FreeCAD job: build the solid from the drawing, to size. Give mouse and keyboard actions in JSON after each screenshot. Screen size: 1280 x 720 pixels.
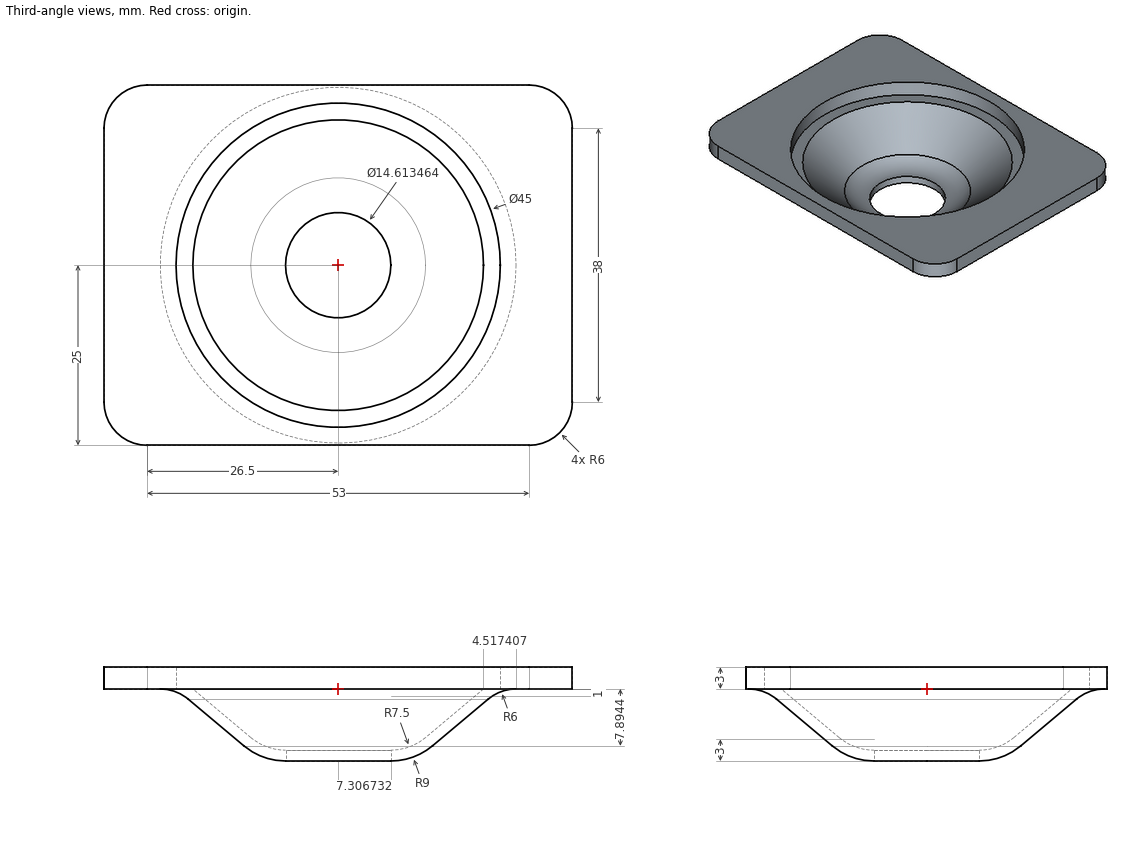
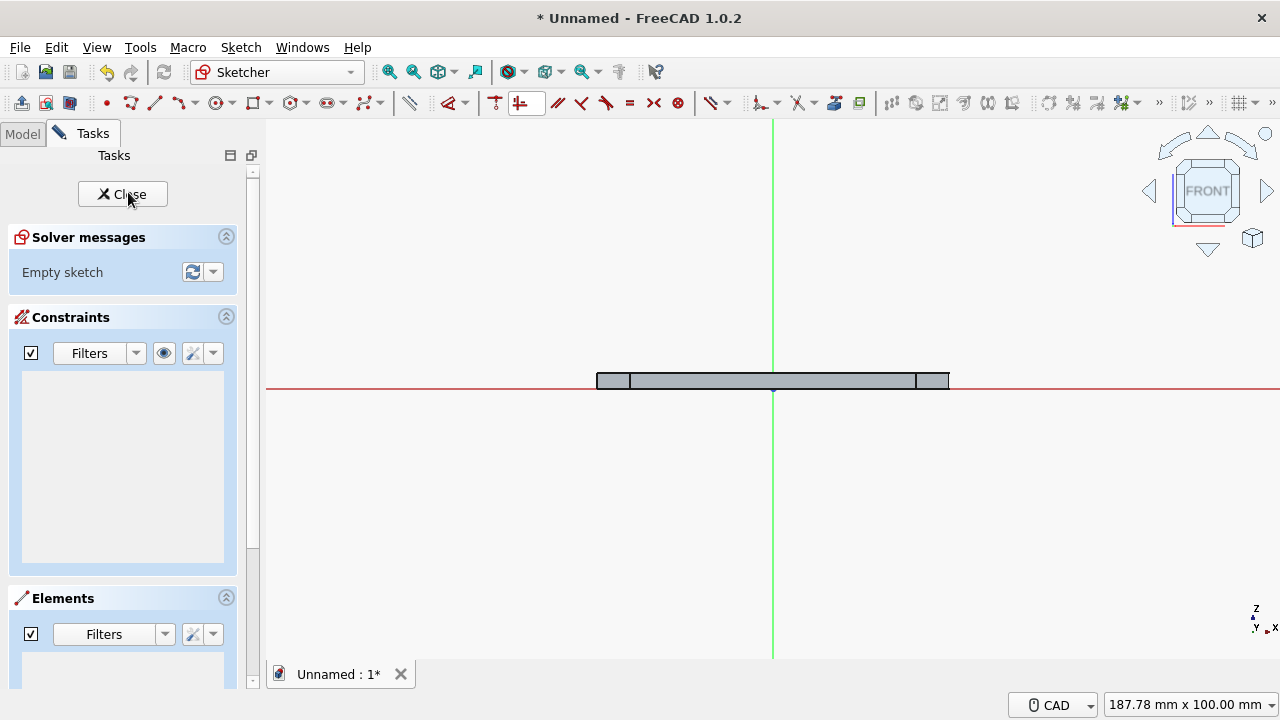
{"action": "left_click", "coordinate": [70, 104]}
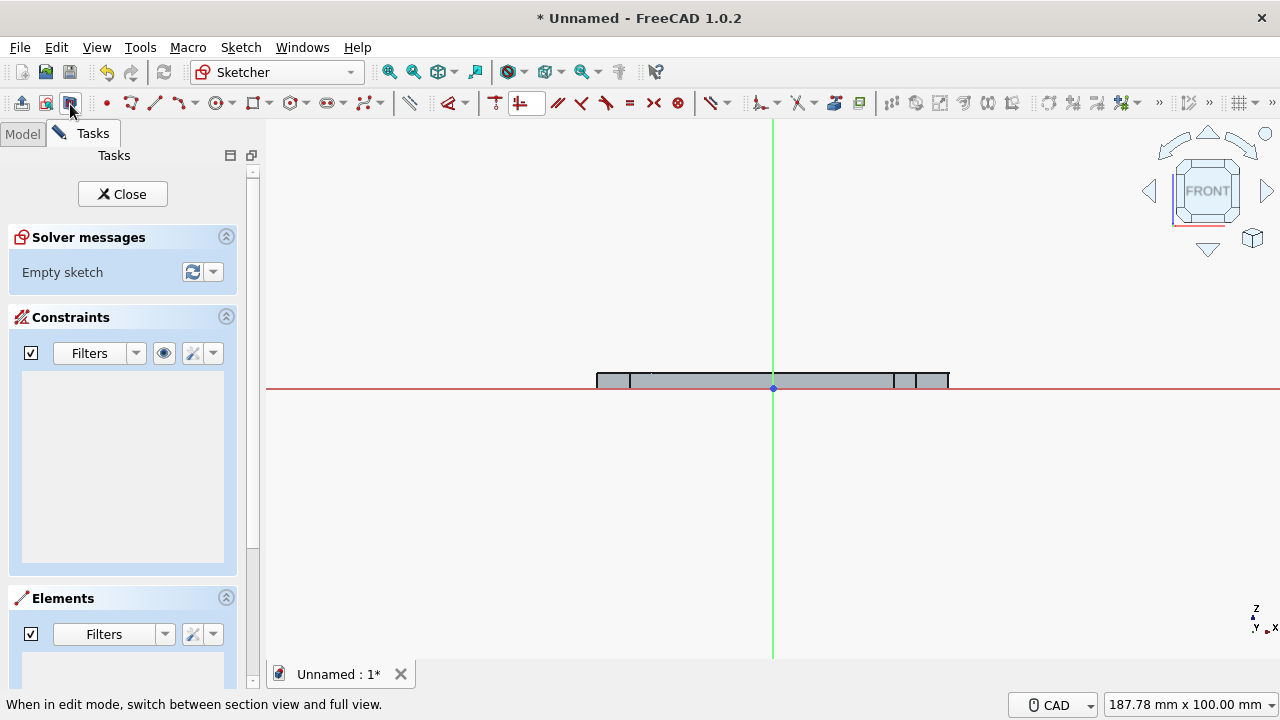
{"action": "scroll", "coordinate": [884, 425], "scroll_direction": "up", "scroll_amount": 7}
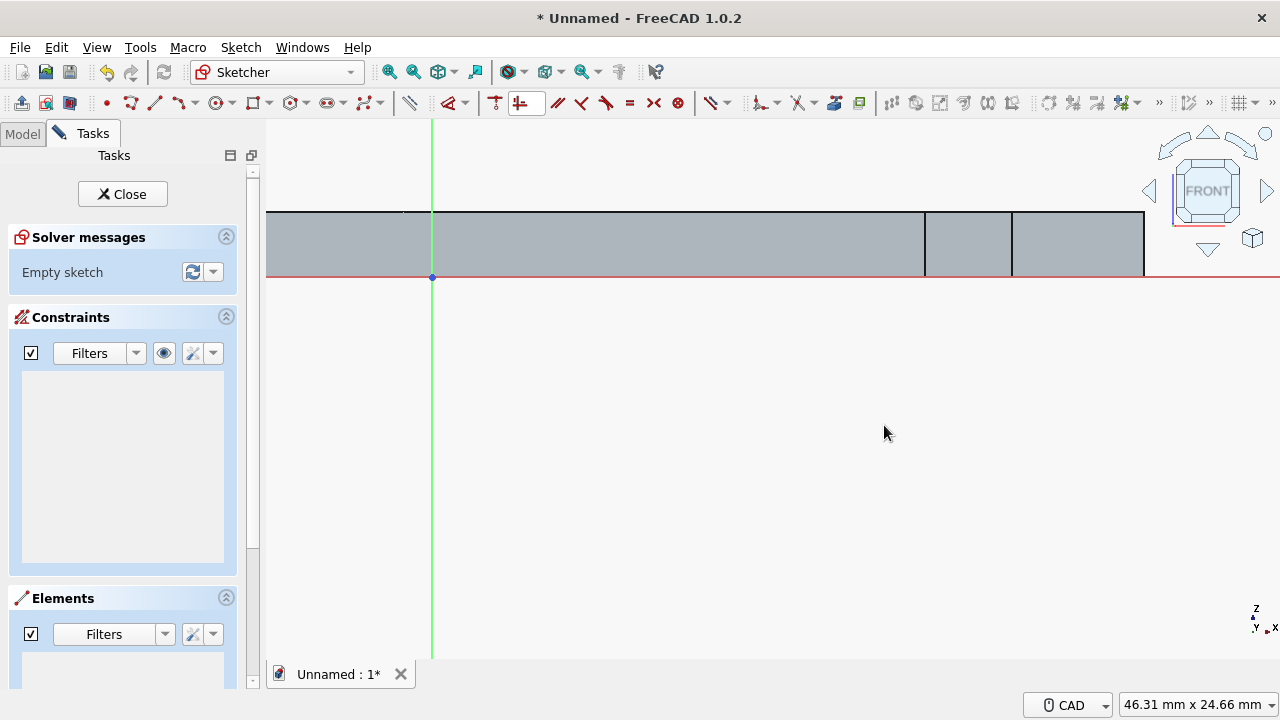
{"action": "key", "text": "g l"}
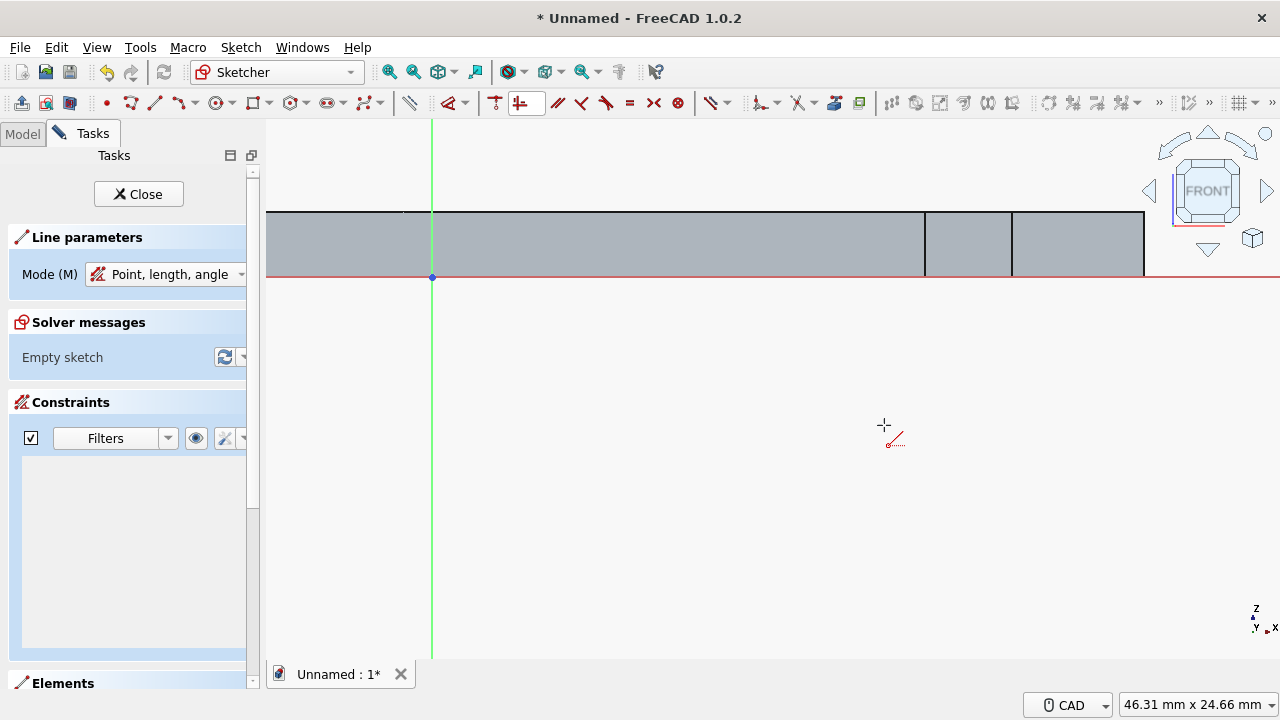
{"action": "left_click", "coordinate": [888, 308]}
{"action": "left_click", "coordinate": [719, 450]}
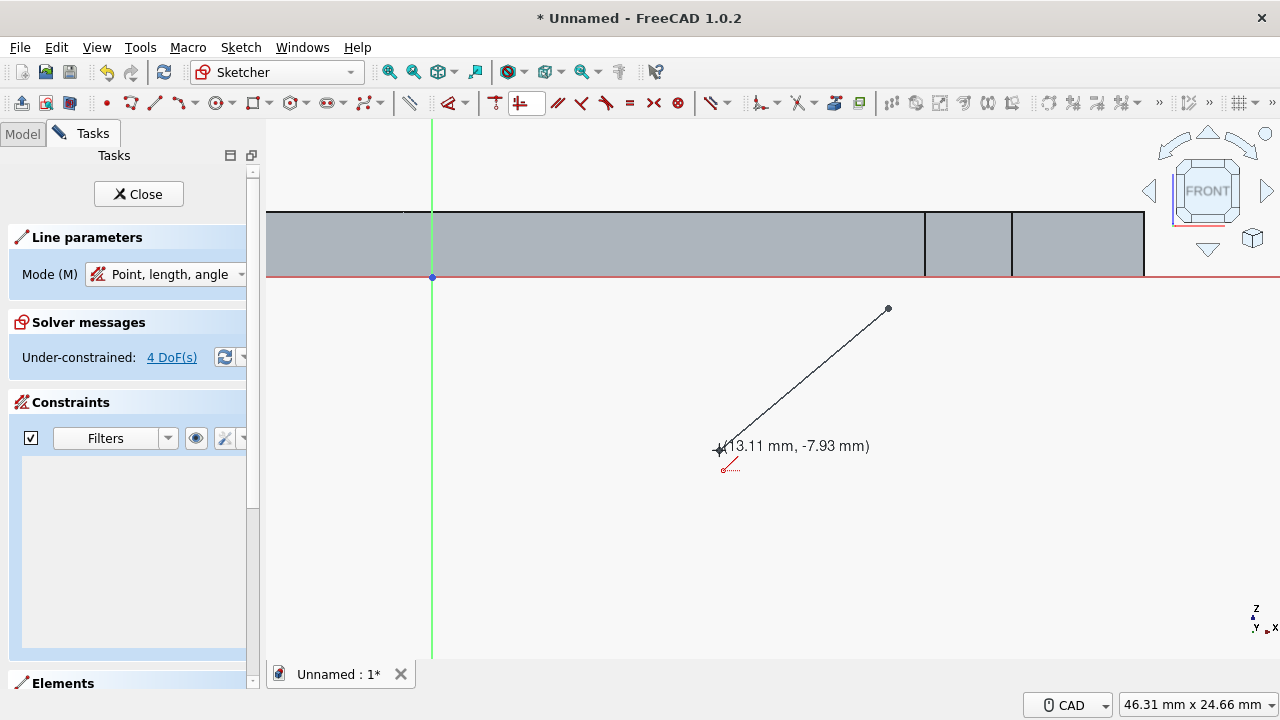
{"action": "key", "text": "g m"}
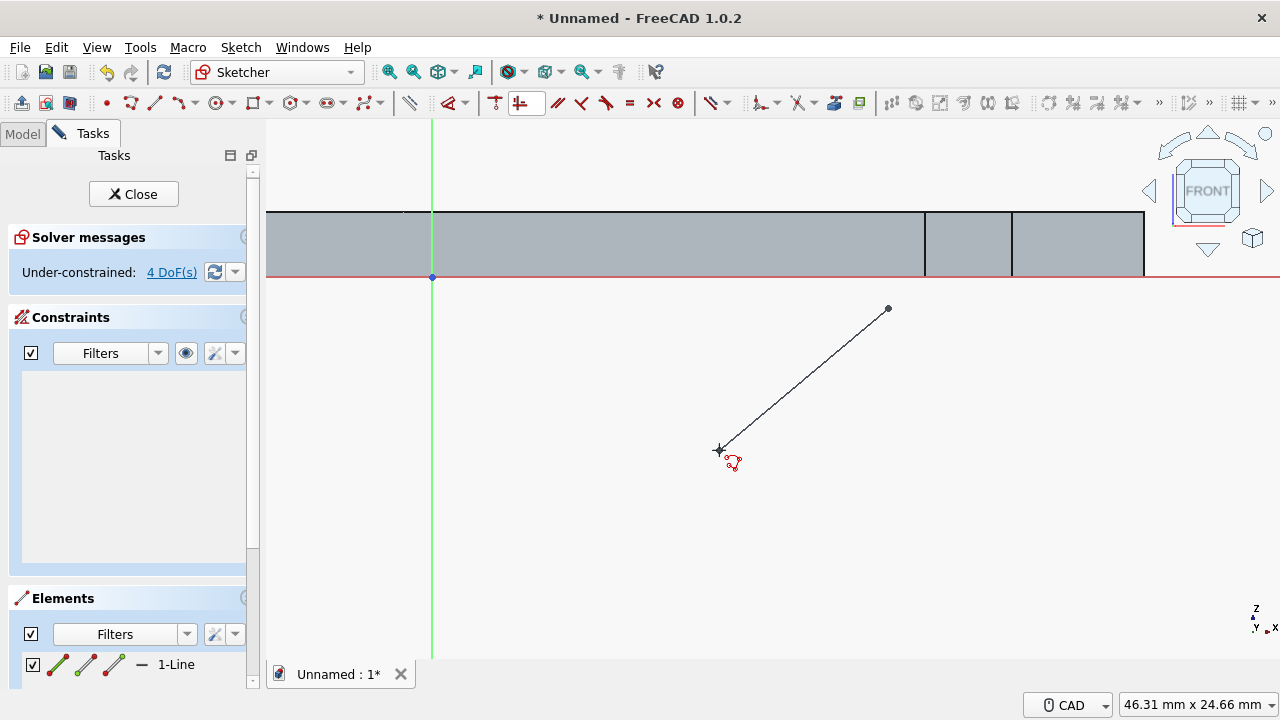
{"action": "left_click", "coordinate": [592, 496]}
{"action": "left_click", "coordinate": [432, 496]}
{"action": "left_click", "coordinate": [441, 463]}
{"action": "left_click", "coordinate": [592, 463]}
{"action": "right_click", "coordinate": [592, 463]}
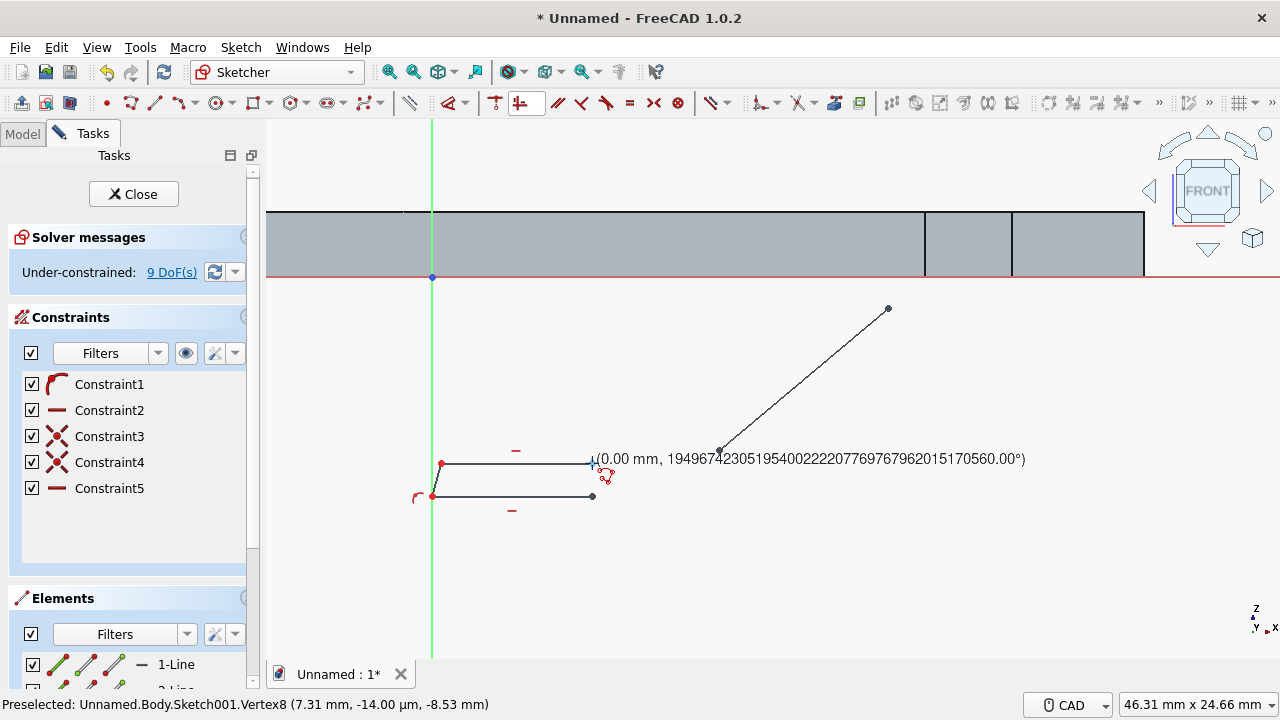
{"action": "left_click", "coordinate": [698, 425]}
{"action": "left_click", "coordinate": [874, 277]}
{"action": "left_click", "coordinate": [973, 286]}
{"action": "right_click", "coordinate": [973, 286]}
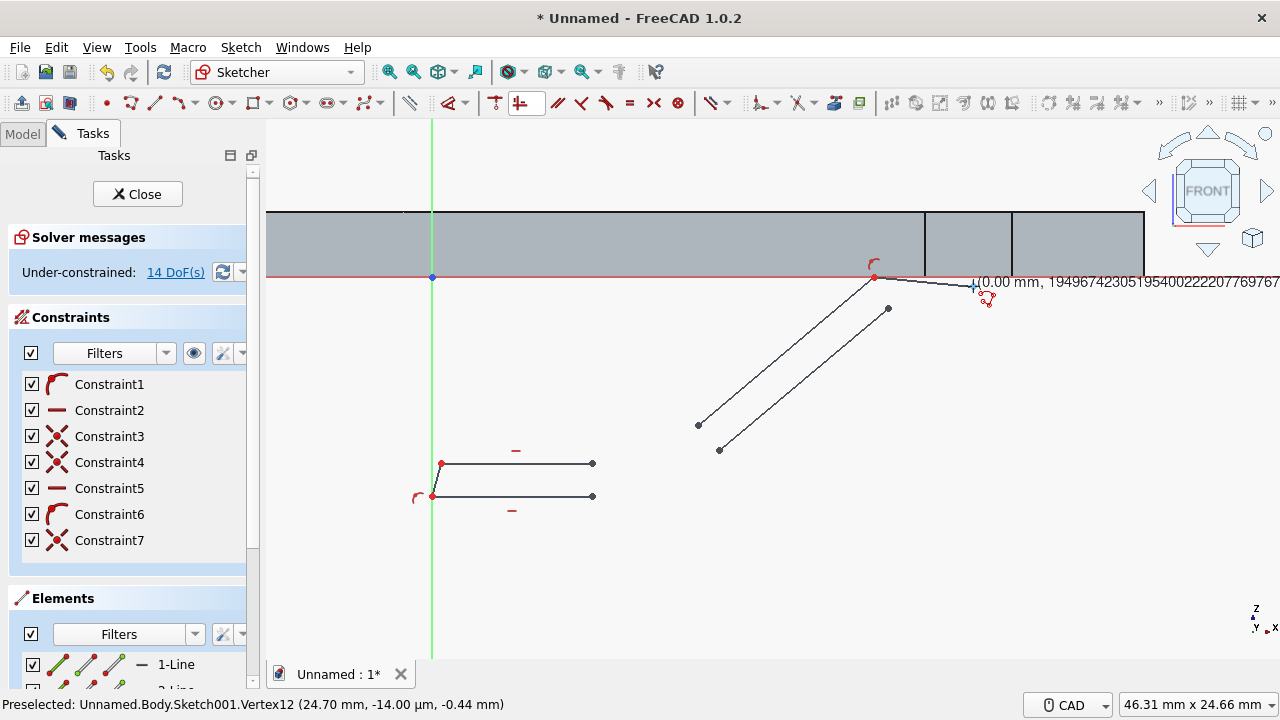
{"action": "left_click", "coordinate": [180, 104]}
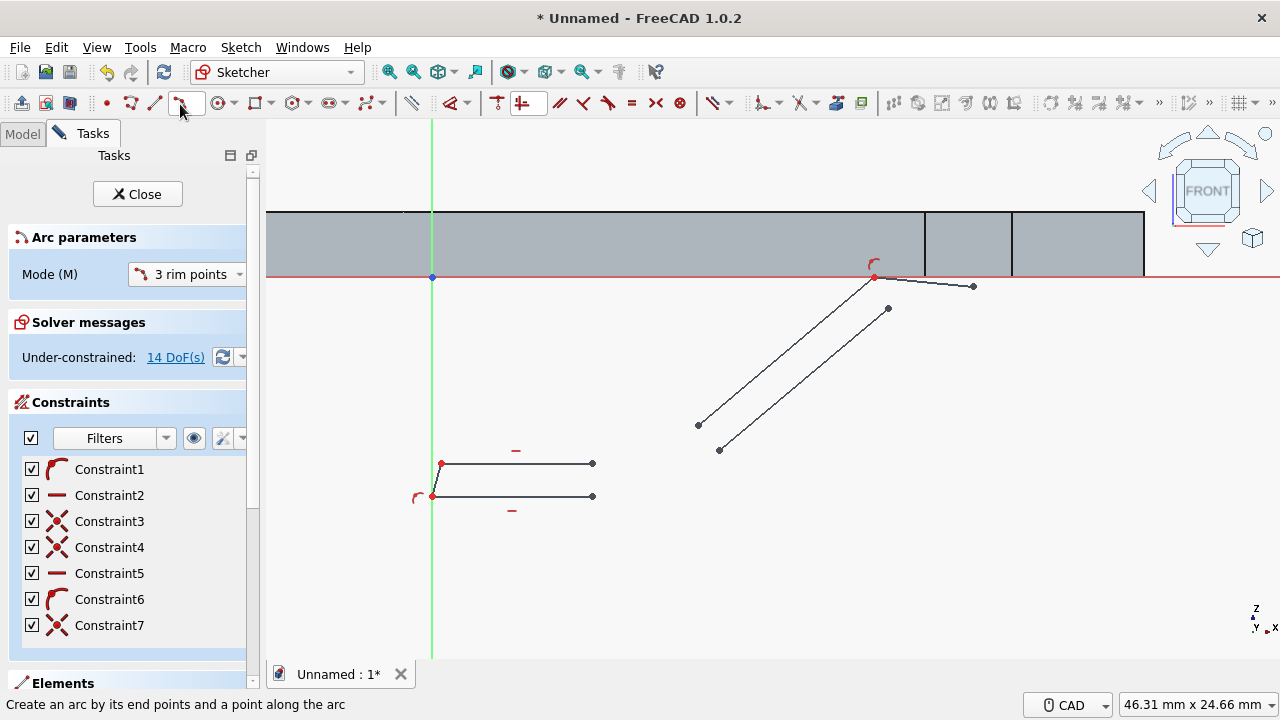
{"action": "left_click", "coordinate": [719, 451]}
{"action": "left_click", "coordinate": [592, 497]}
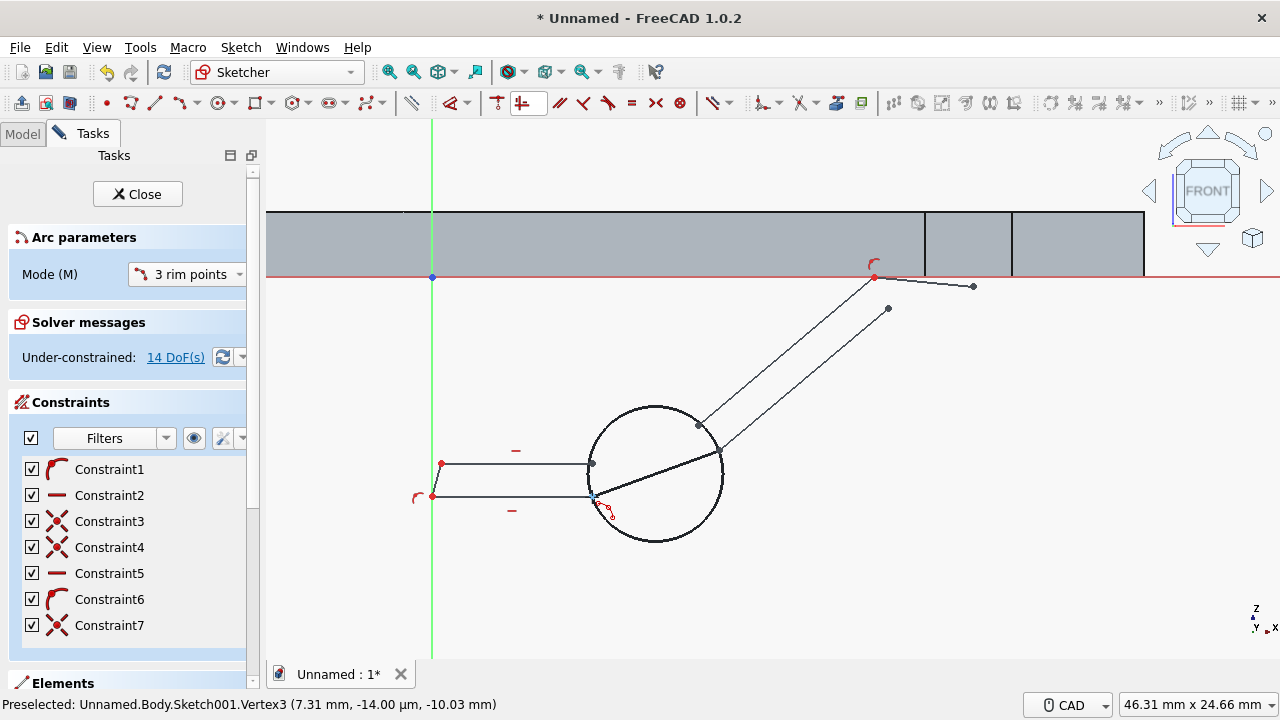
{"action": "scroll", "coordinate": [659, 484], "scroll_direction": "up", "scroll_amount": 2}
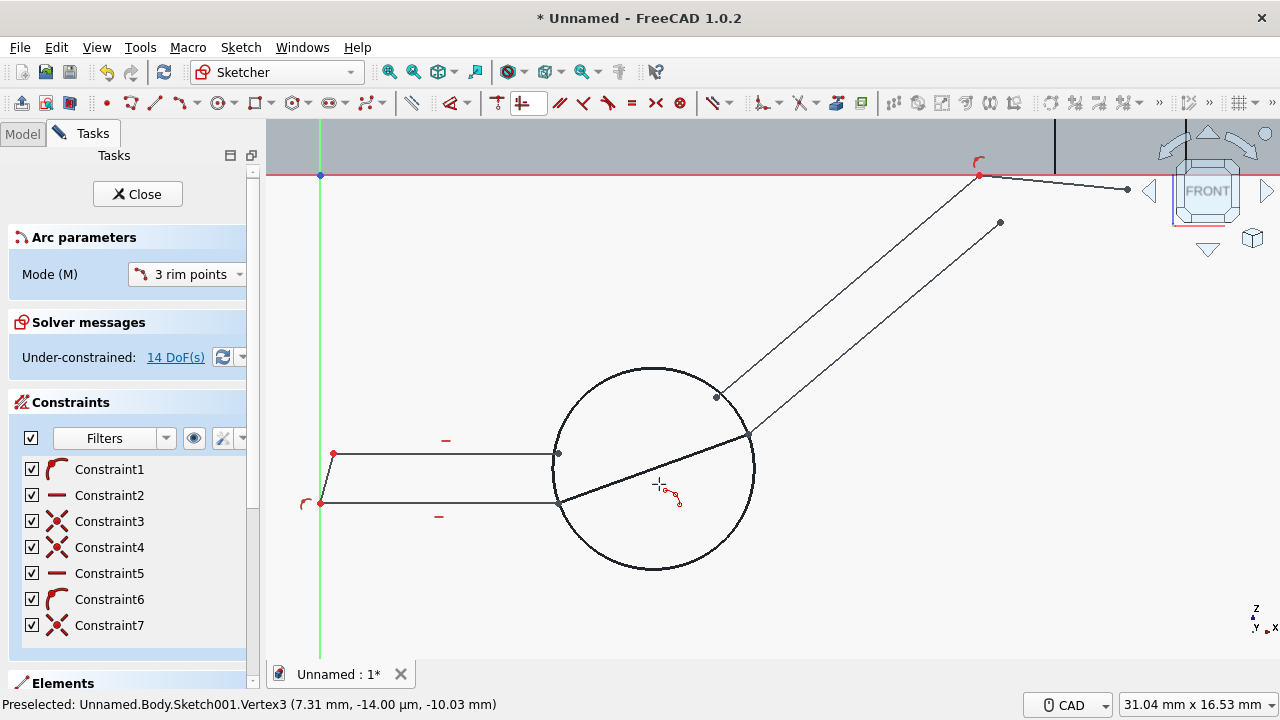
{"action": "left_click", "coordinate": [659, 484]}